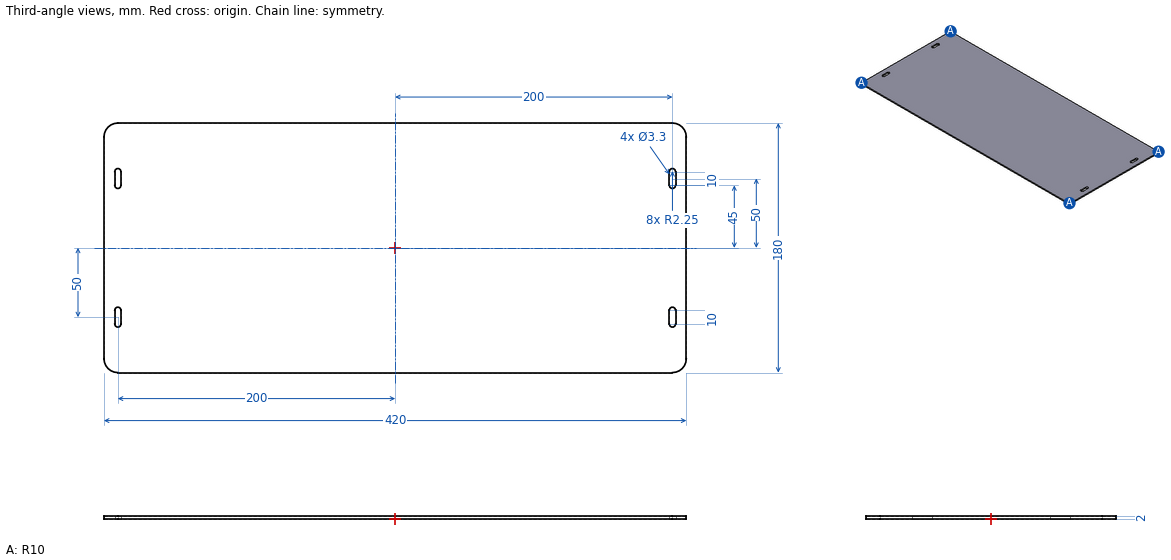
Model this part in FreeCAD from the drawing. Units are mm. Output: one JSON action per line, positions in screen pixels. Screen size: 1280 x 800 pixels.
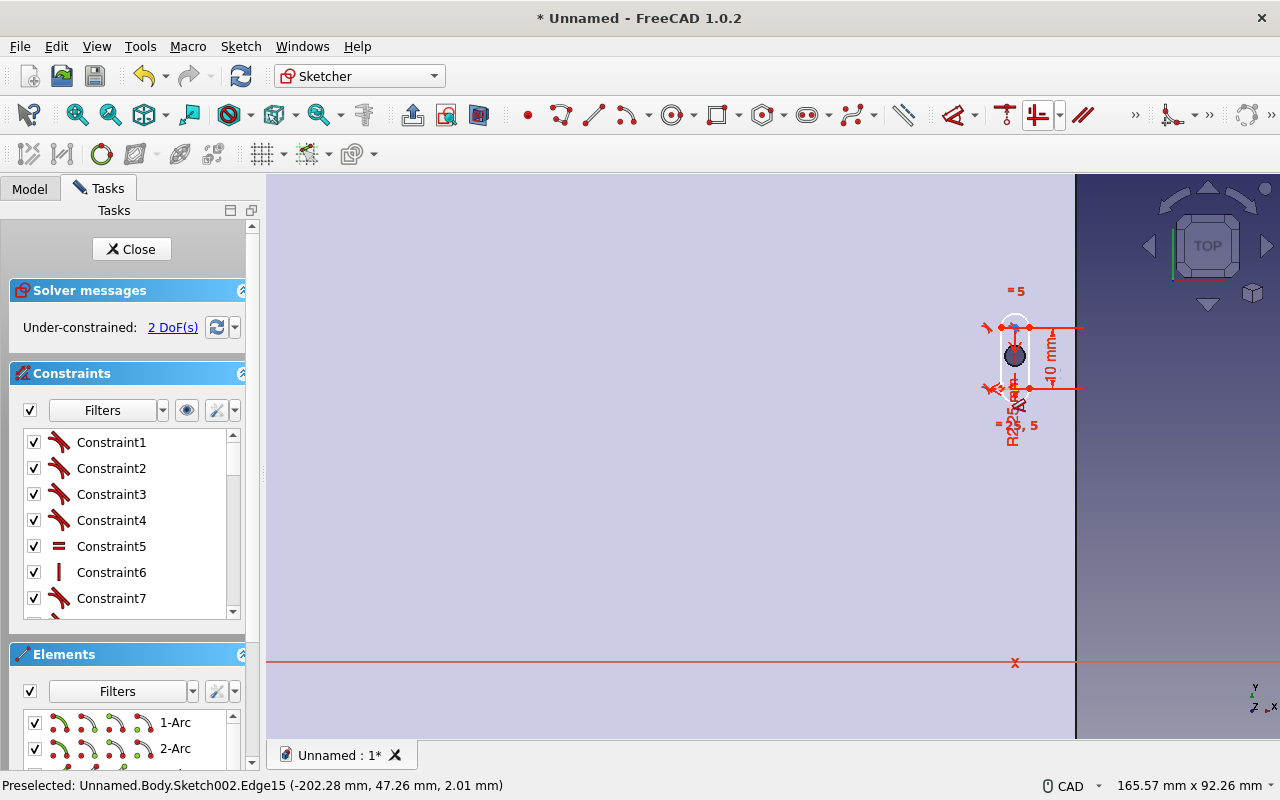
{"action": "left_click", "coordinate": [1001, 389]}
{"action": "left_click", "coordinate": [1035, 525]}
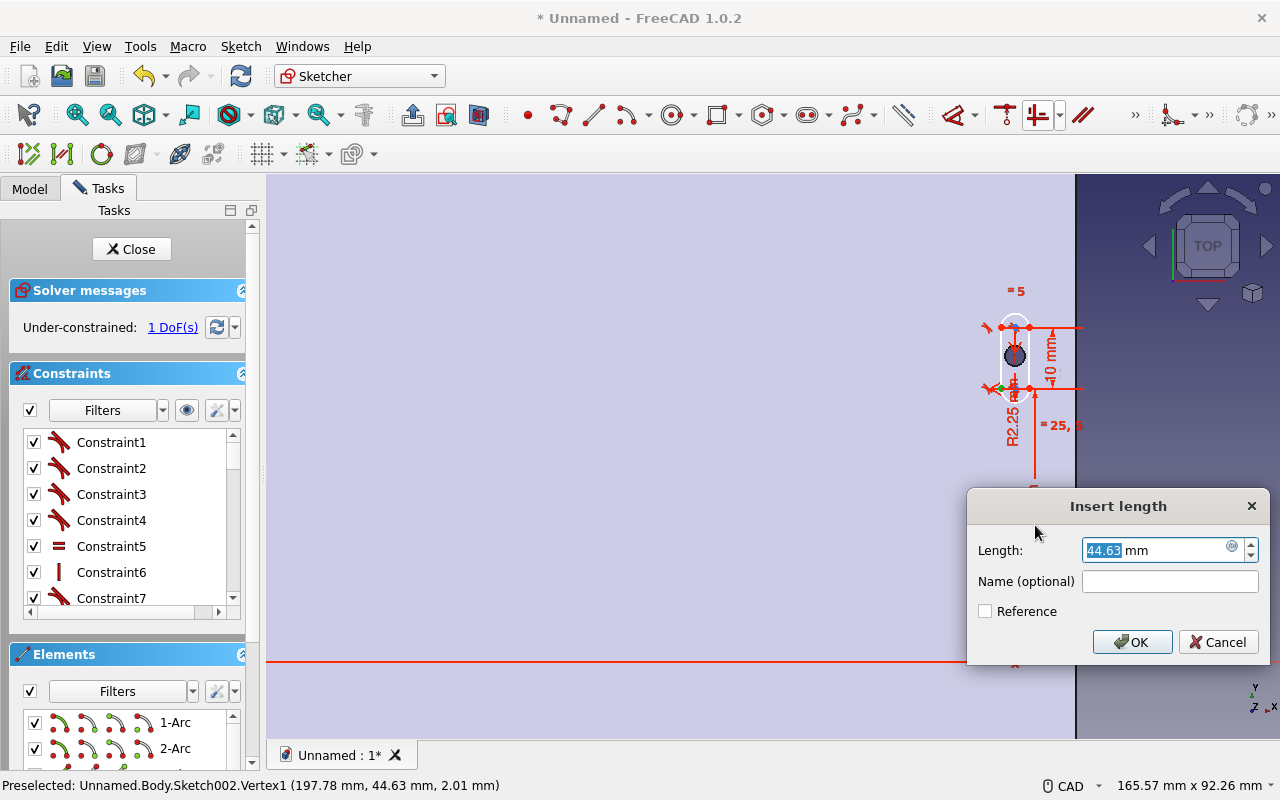
{"action": "type", "text": "45"}
{"action": "key", "text": "Return"}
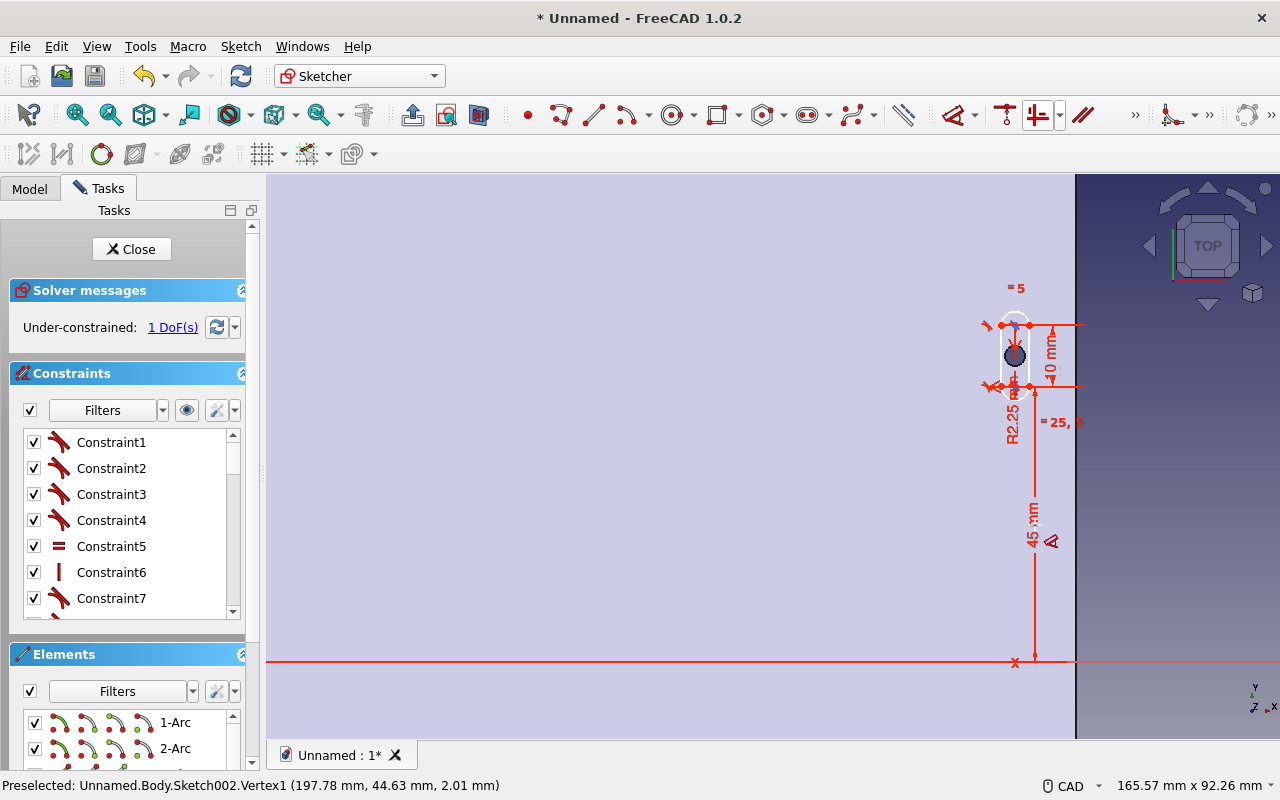
{"action": "left_click", "coordinate": [1015, 387]}
{"action": "left_click", "coordinate": [655, 353]}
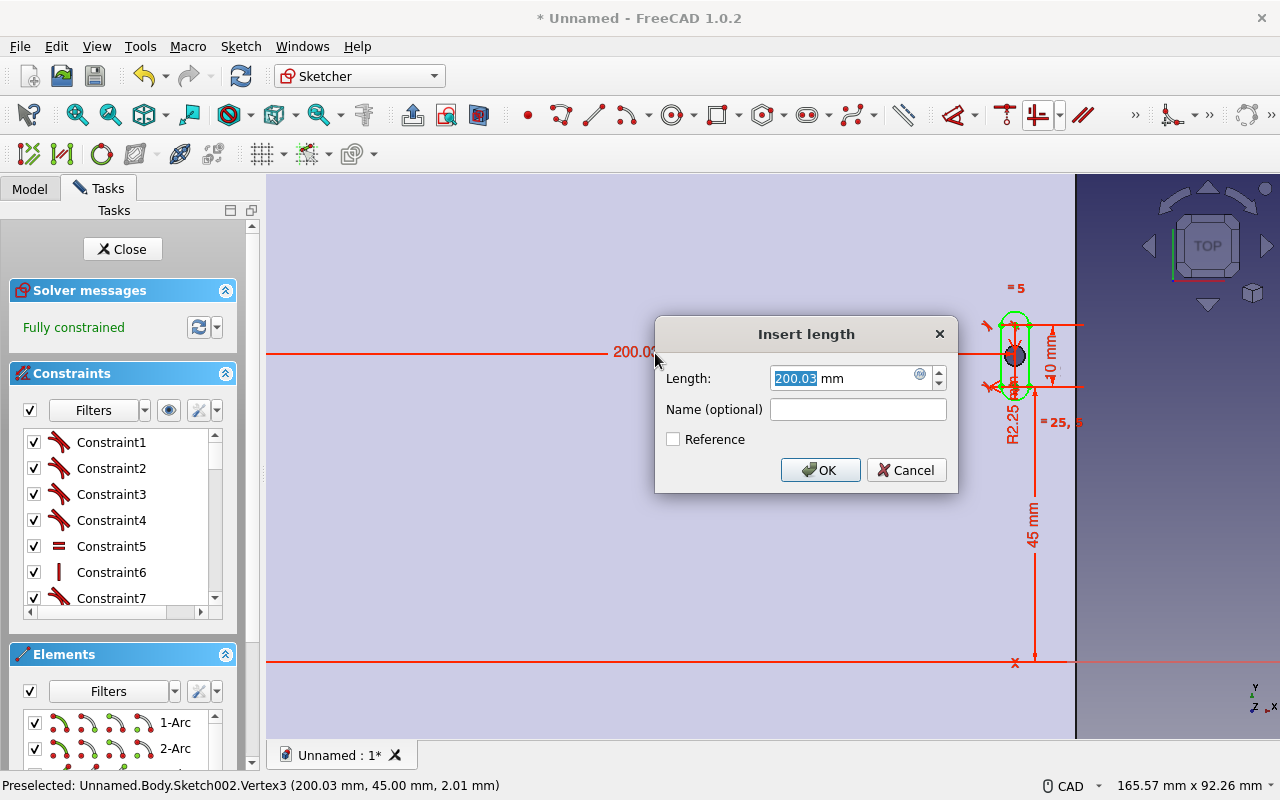
{"action": "type", "text": "200"}
{"action": "key", "text": "Return"}
{"action": "key", "text": "Escape"}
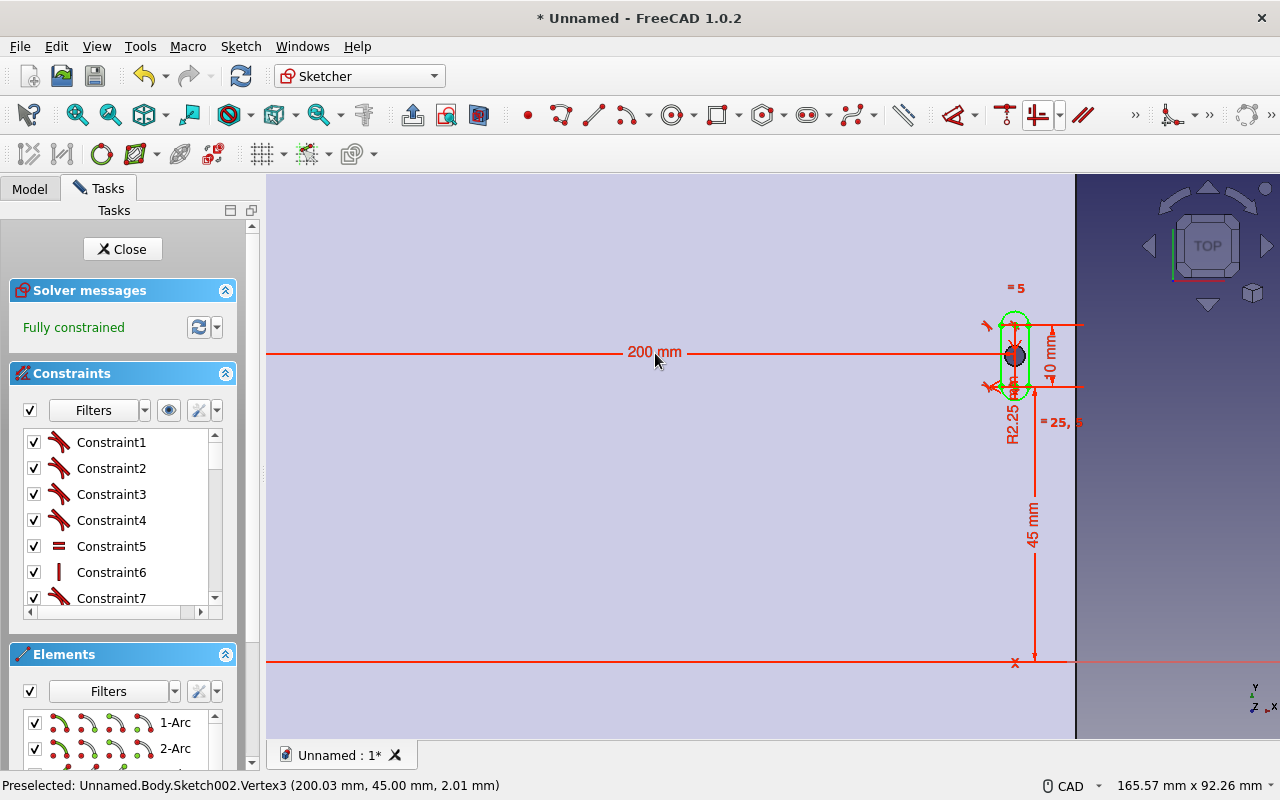
{"action": "left_click", "coordinate": [123, 249]}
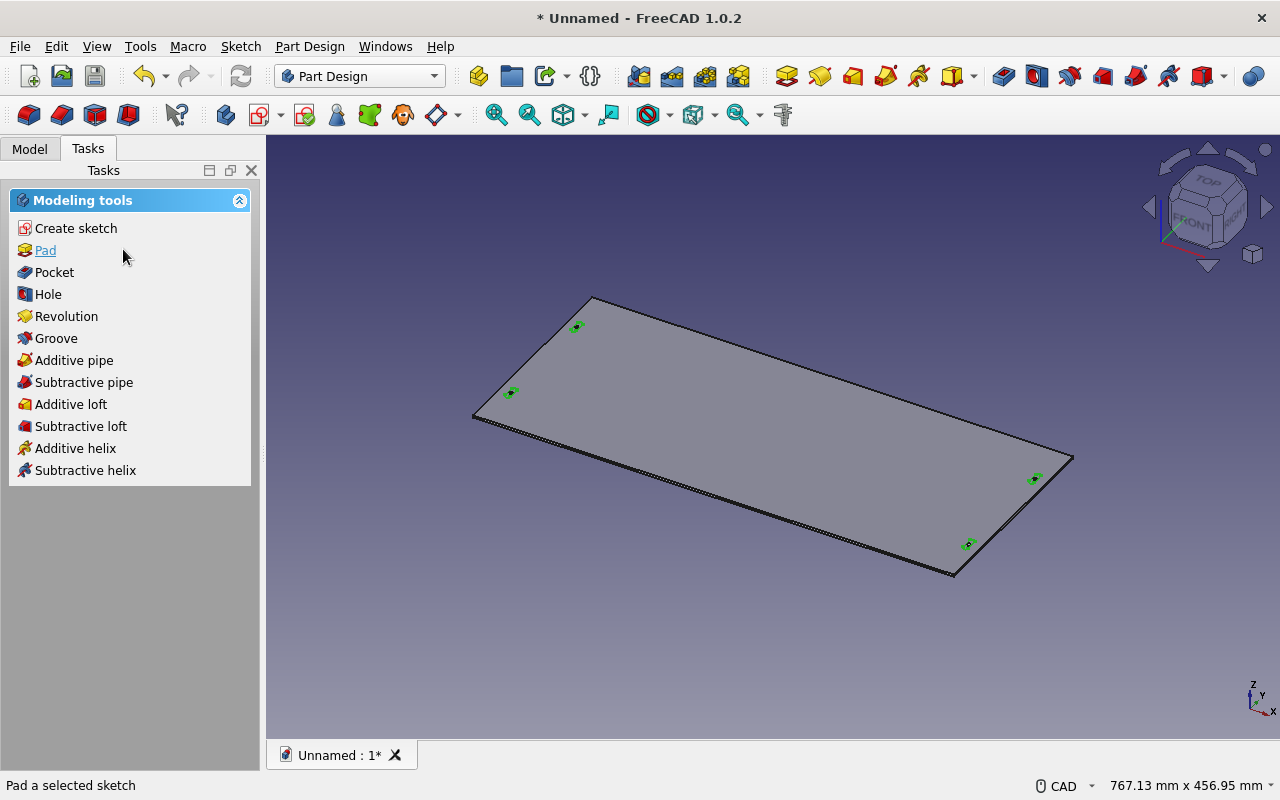
{"action": "left_click", "coordinate": [1004, 76]}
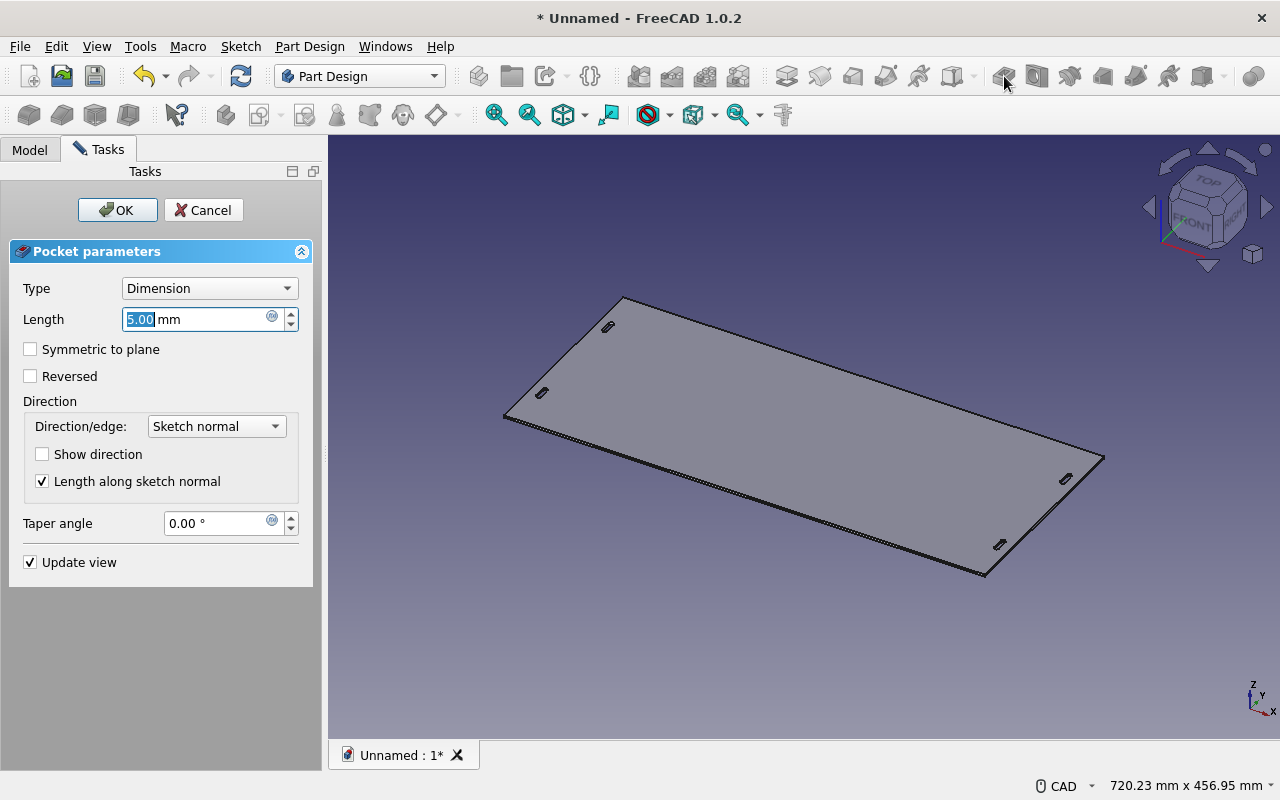
{"action": "type", "text": "10"}
{"action": "key", "text": "Tab"}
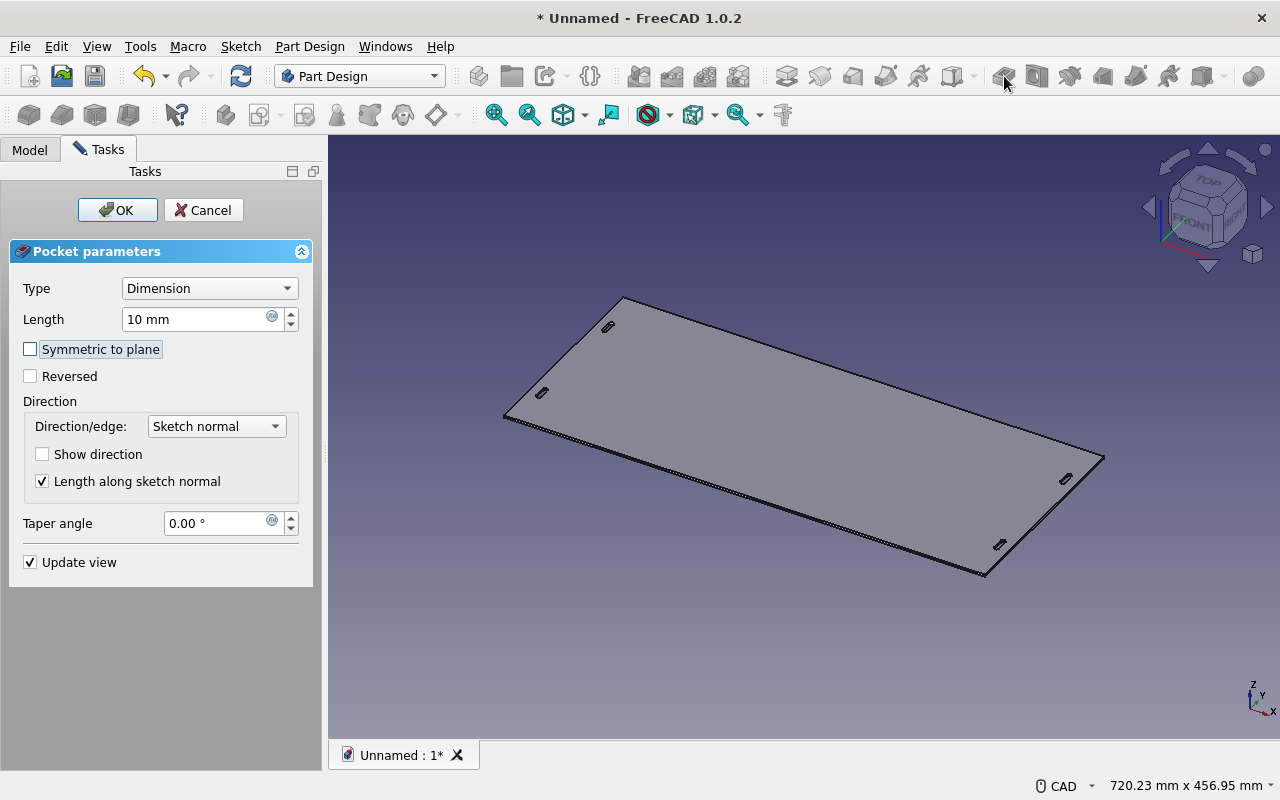
{"action": "left_click", "coordinate": [118, 210]}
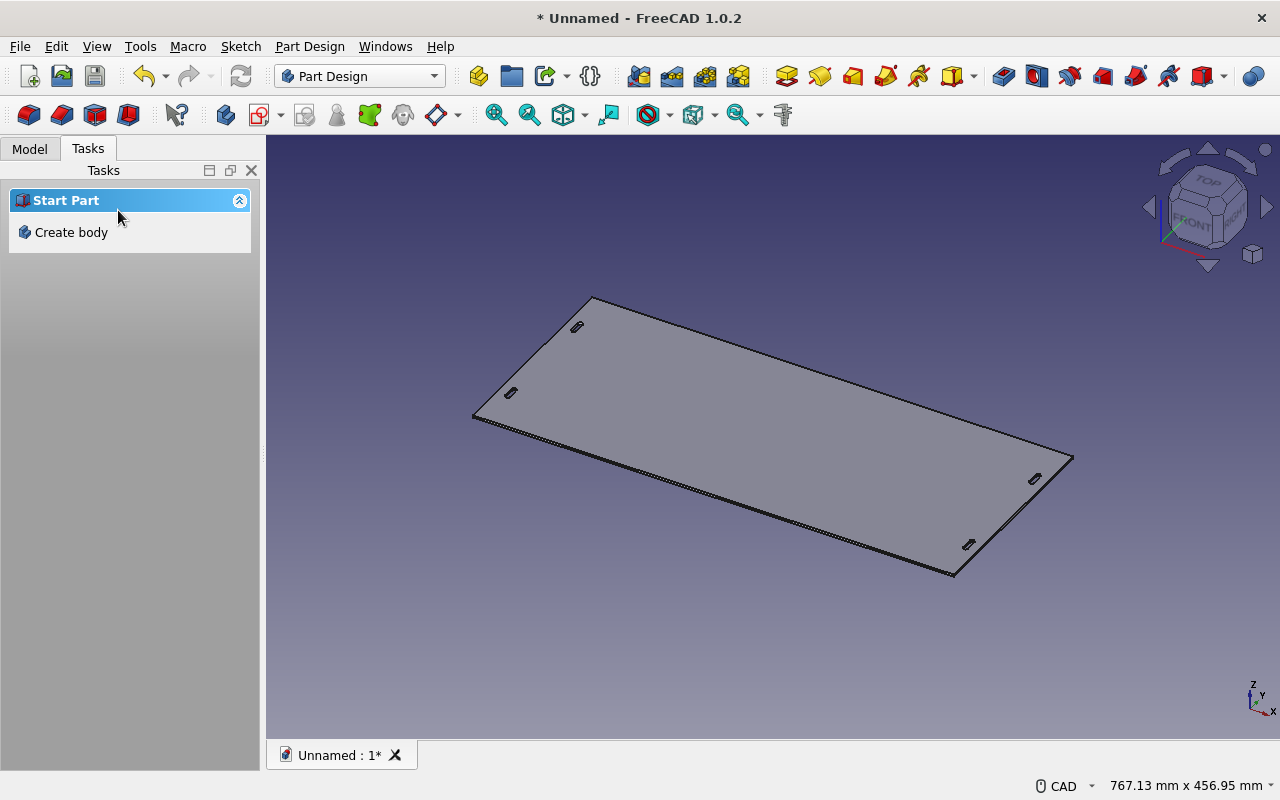
{"action": "scroll", "coordinate": [954, 575], "scroll_direction": "up", "scroll_amount": 14}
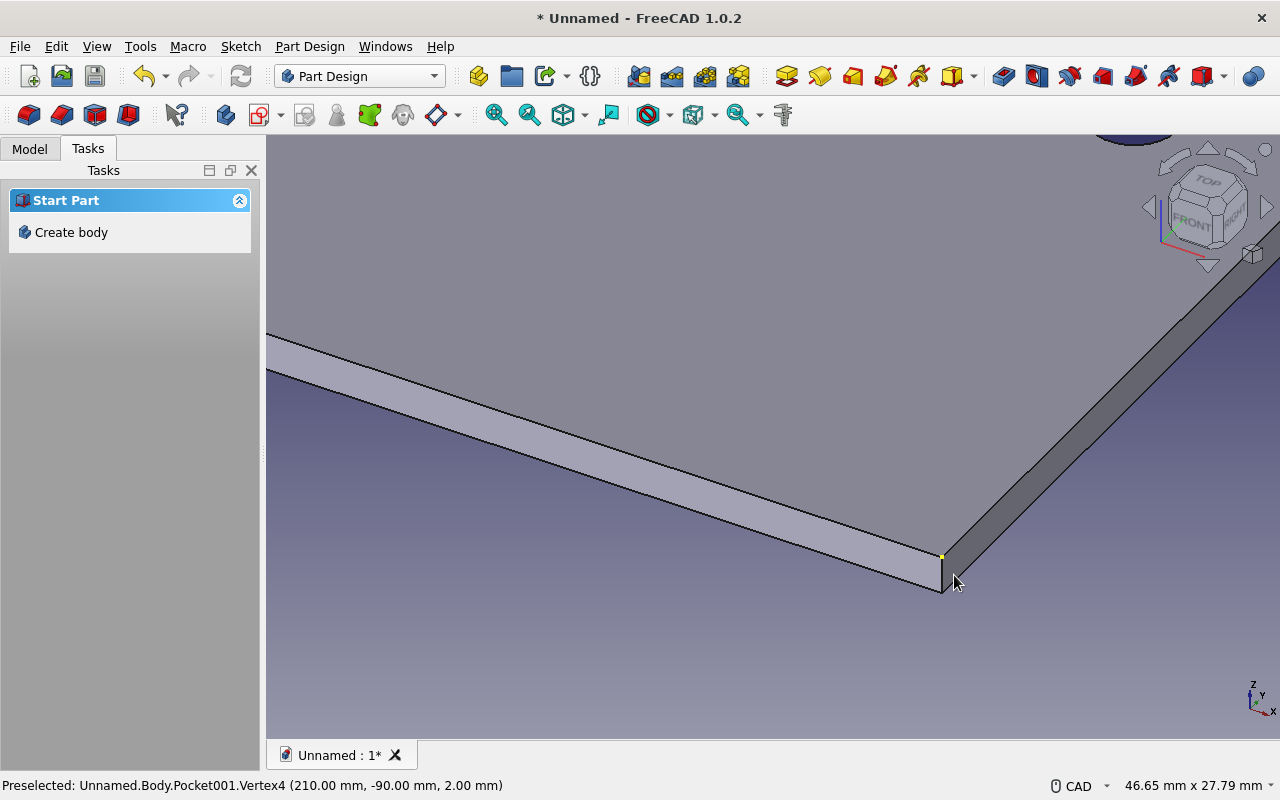
{"action": "left_click", "coordinate": [942, 574]}